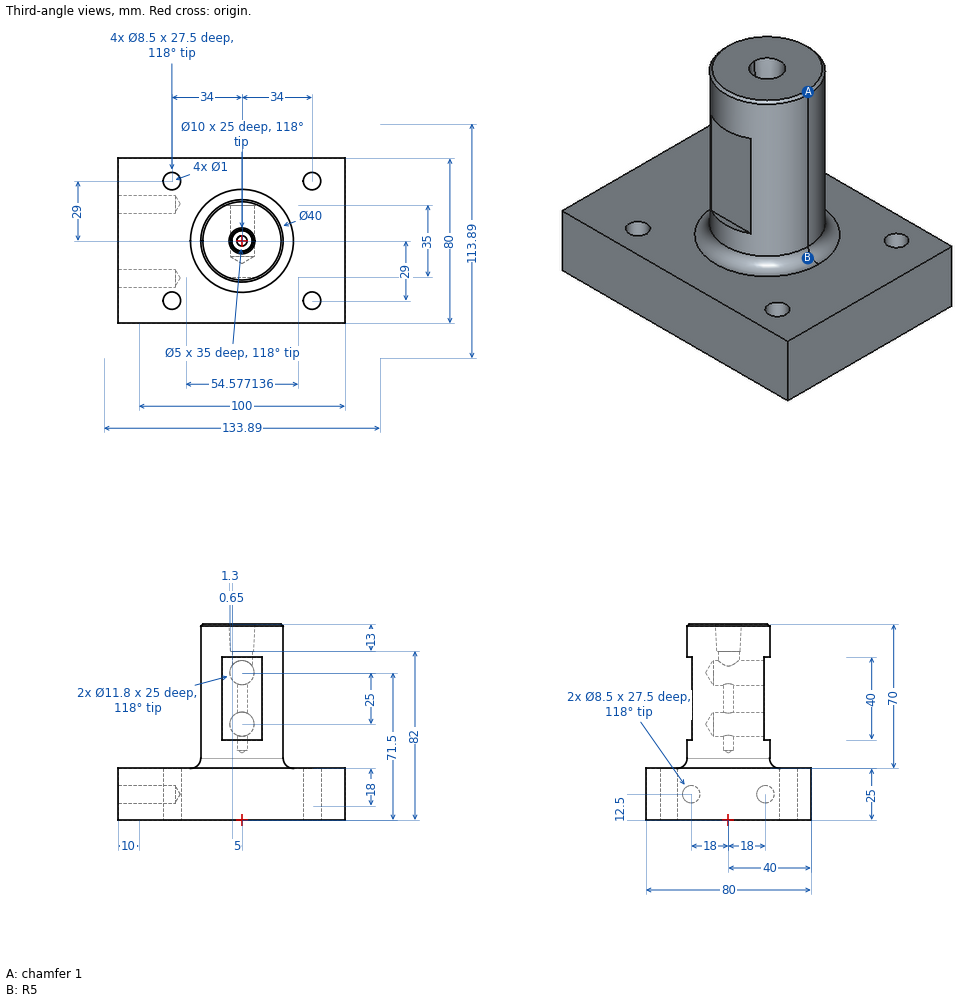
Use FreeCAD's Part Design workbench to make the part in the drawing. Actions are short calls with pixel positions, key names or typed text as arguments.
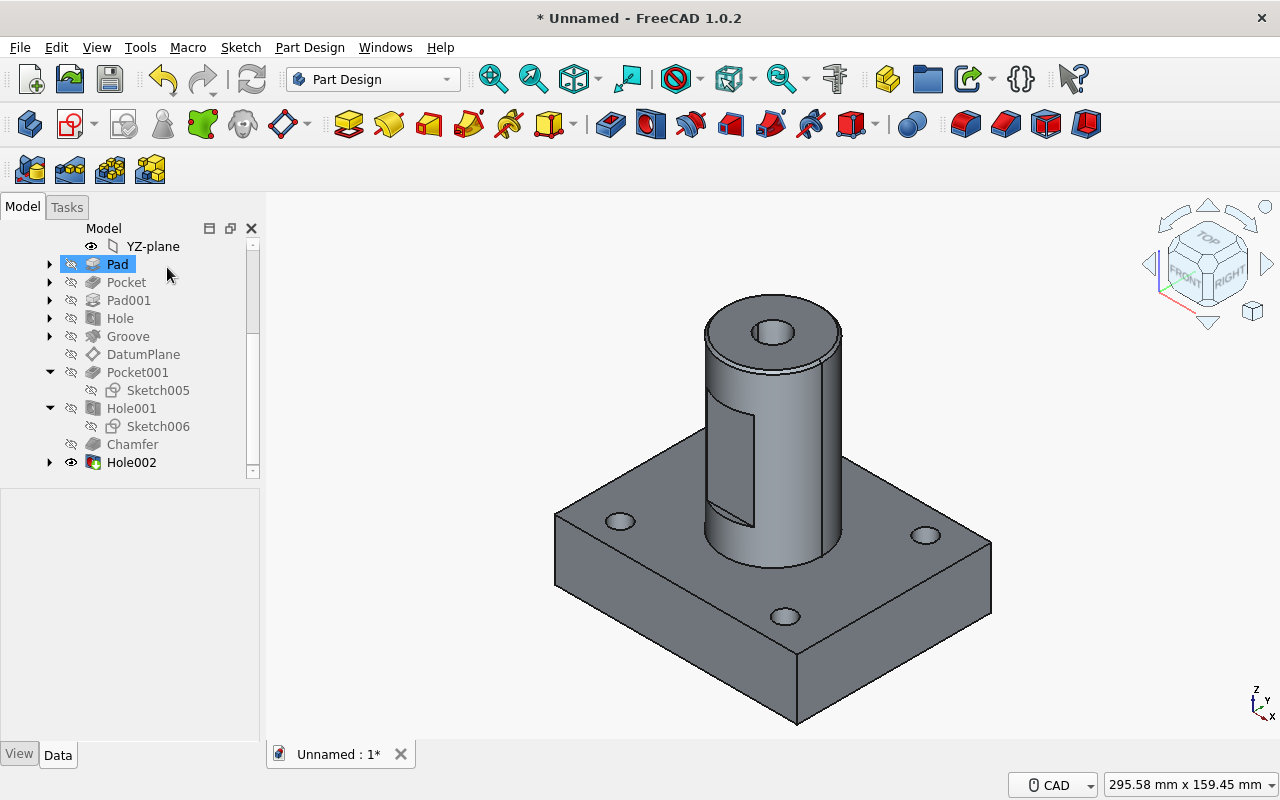
key(1)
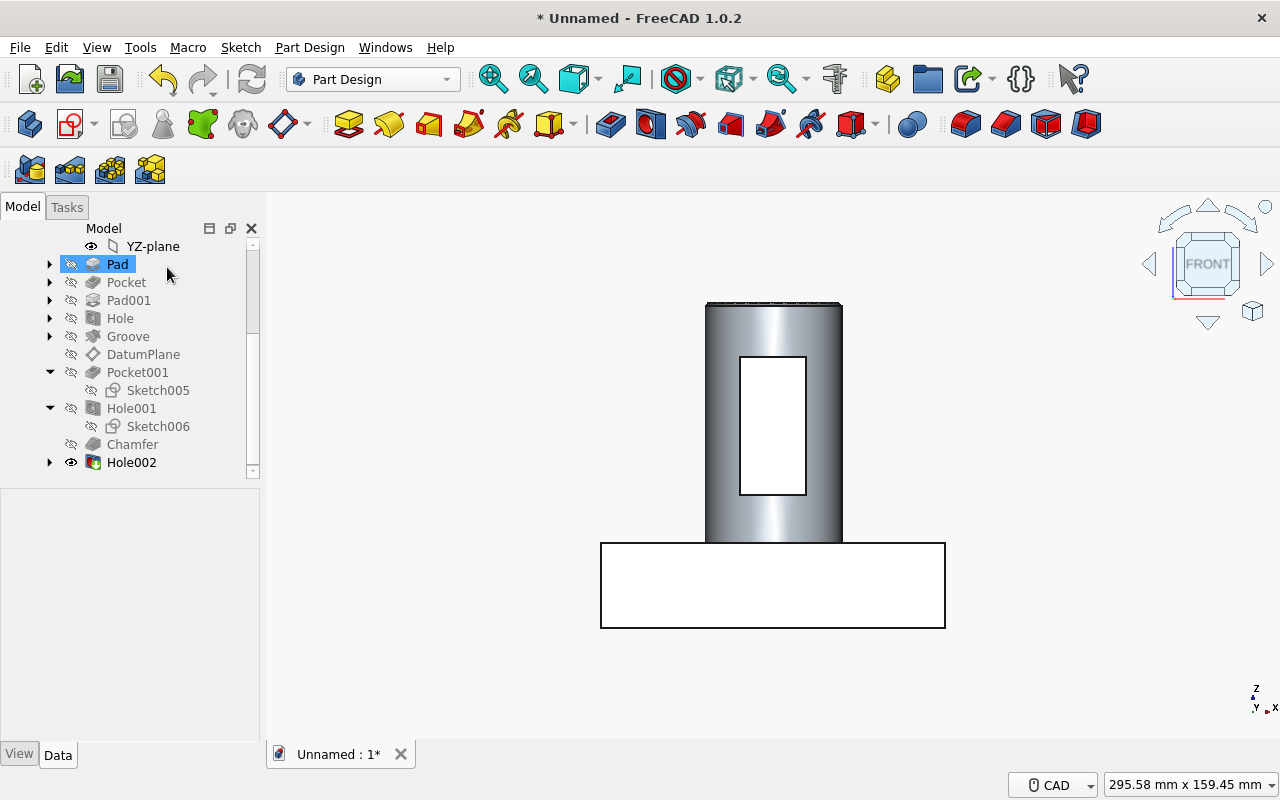
key(3)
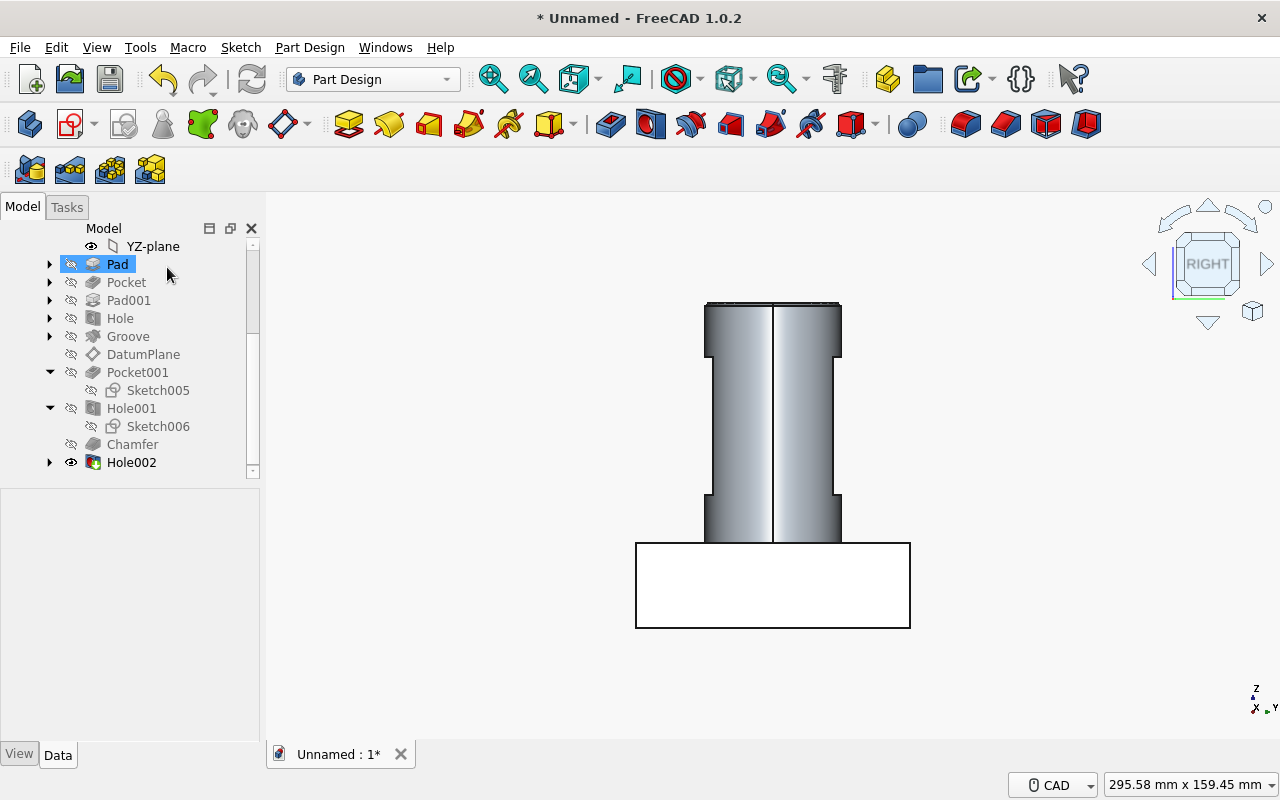
key(5)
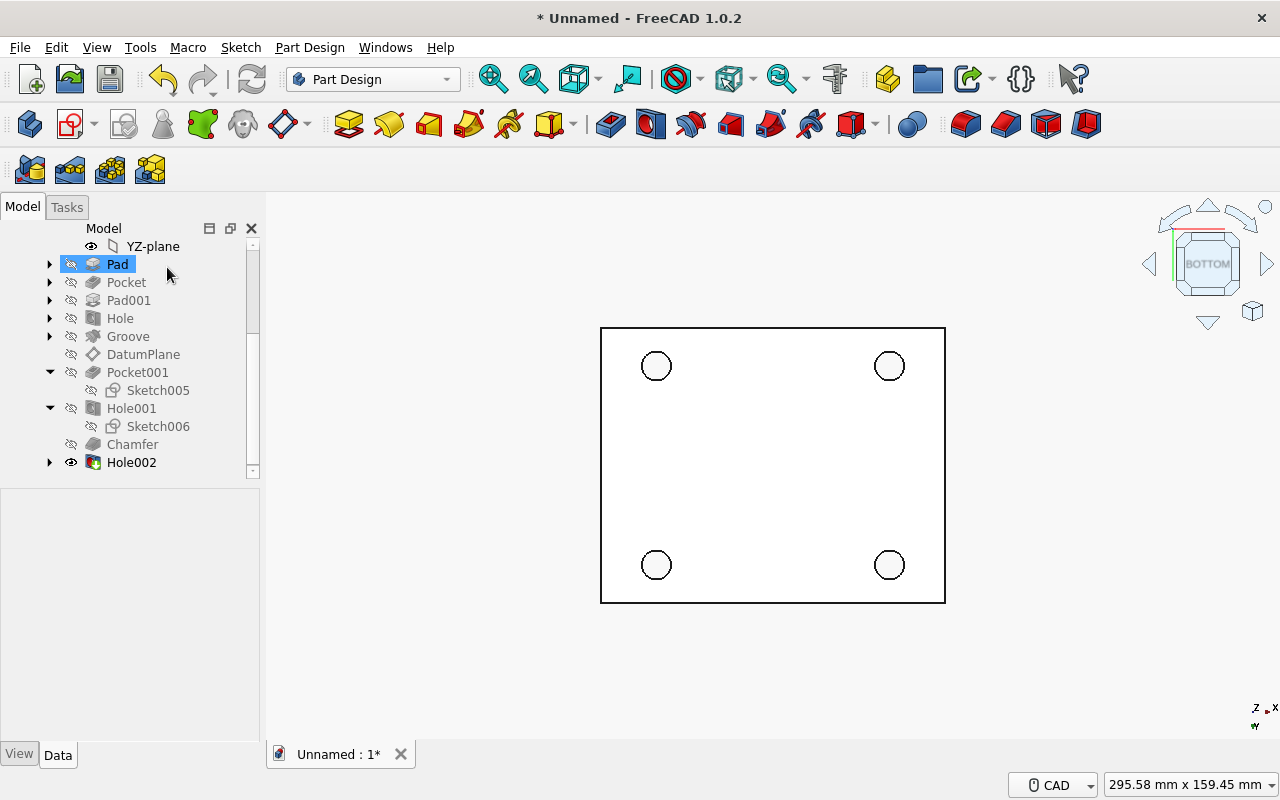
key(4)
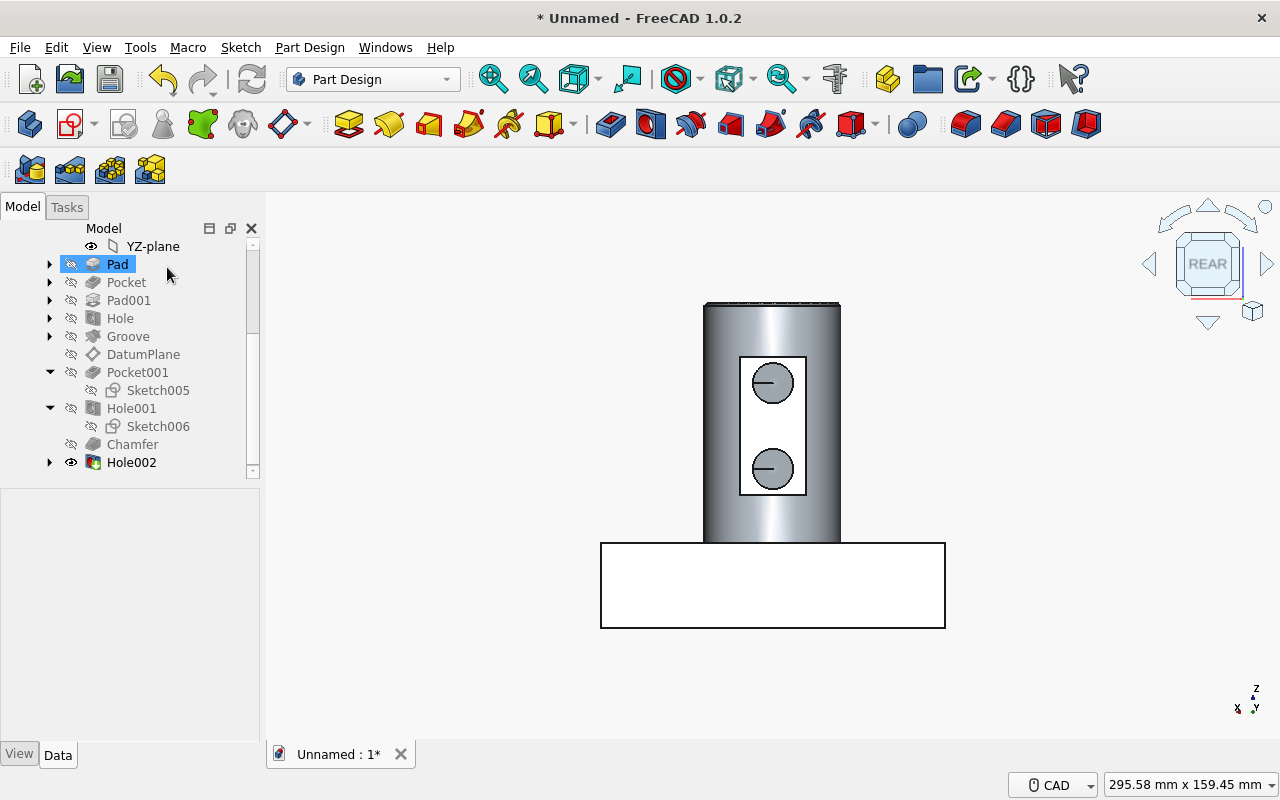
key(6)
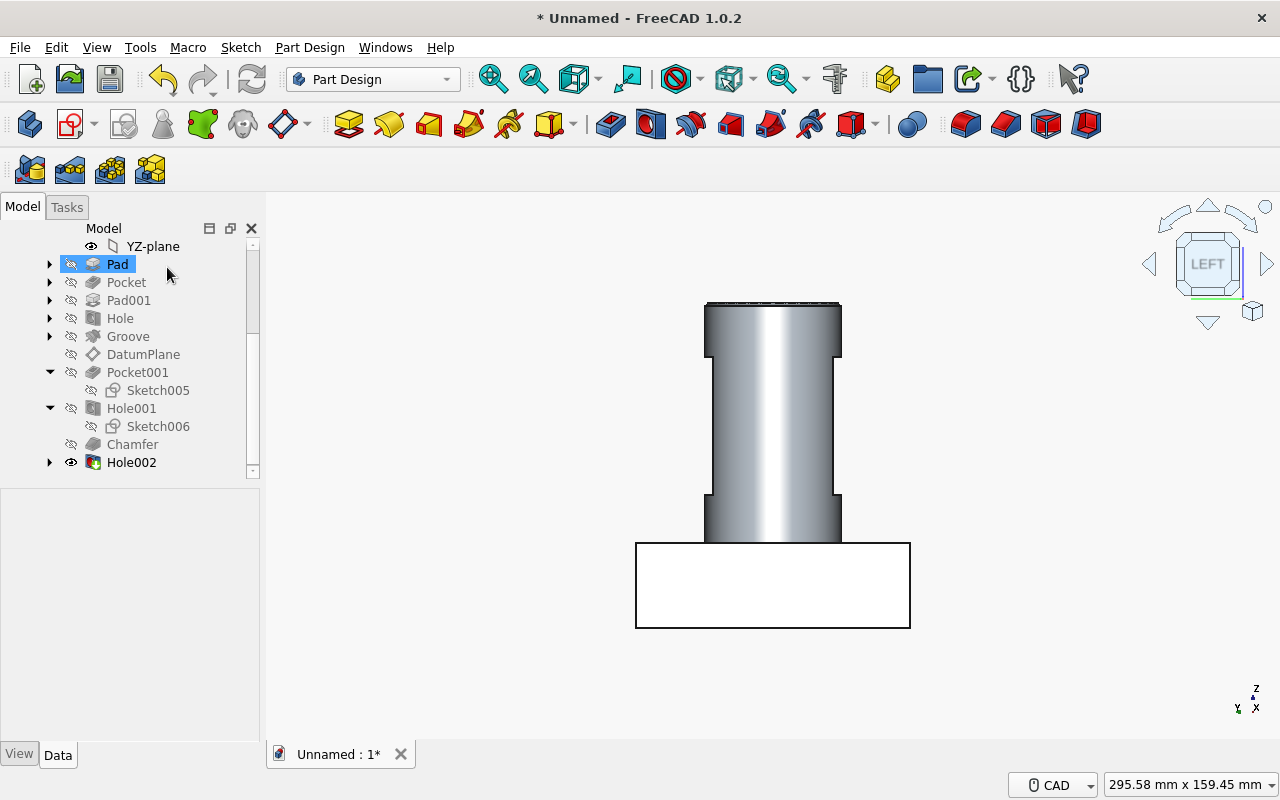
key(v)
key(3)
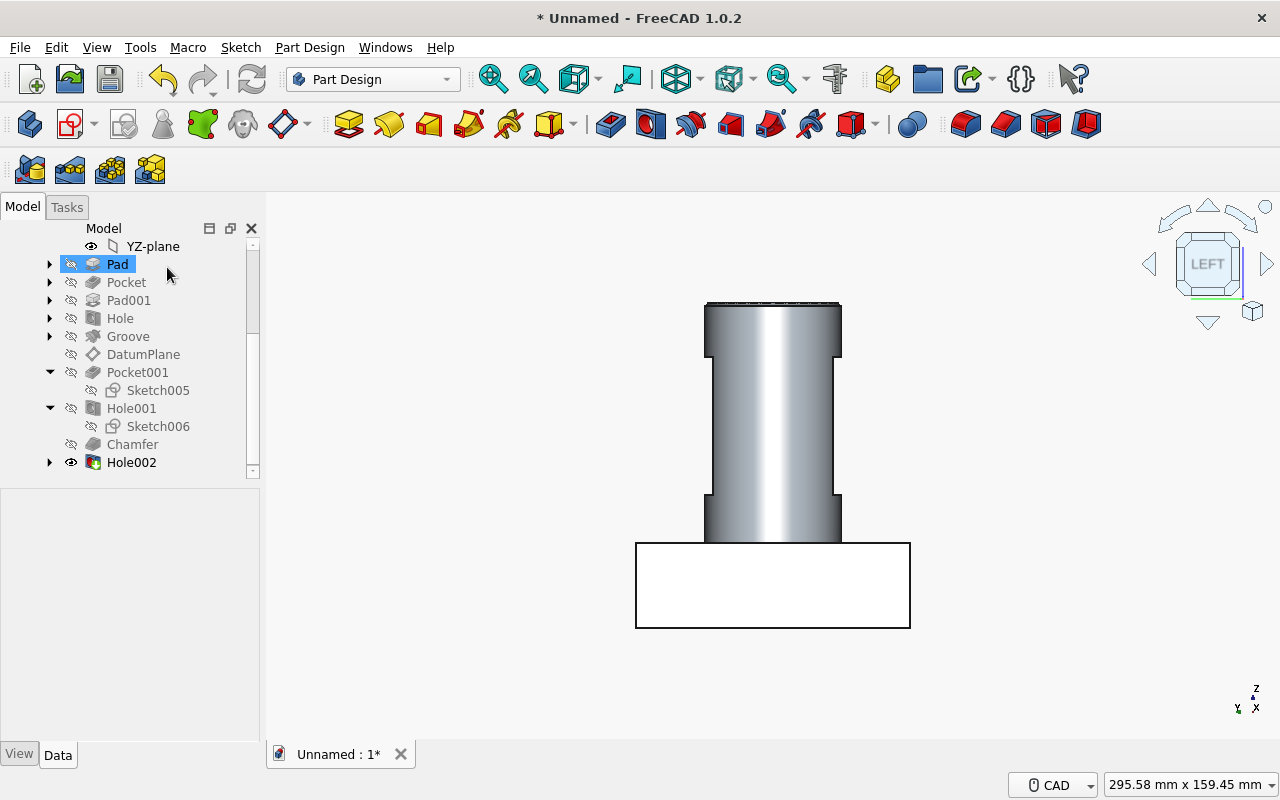
key(0)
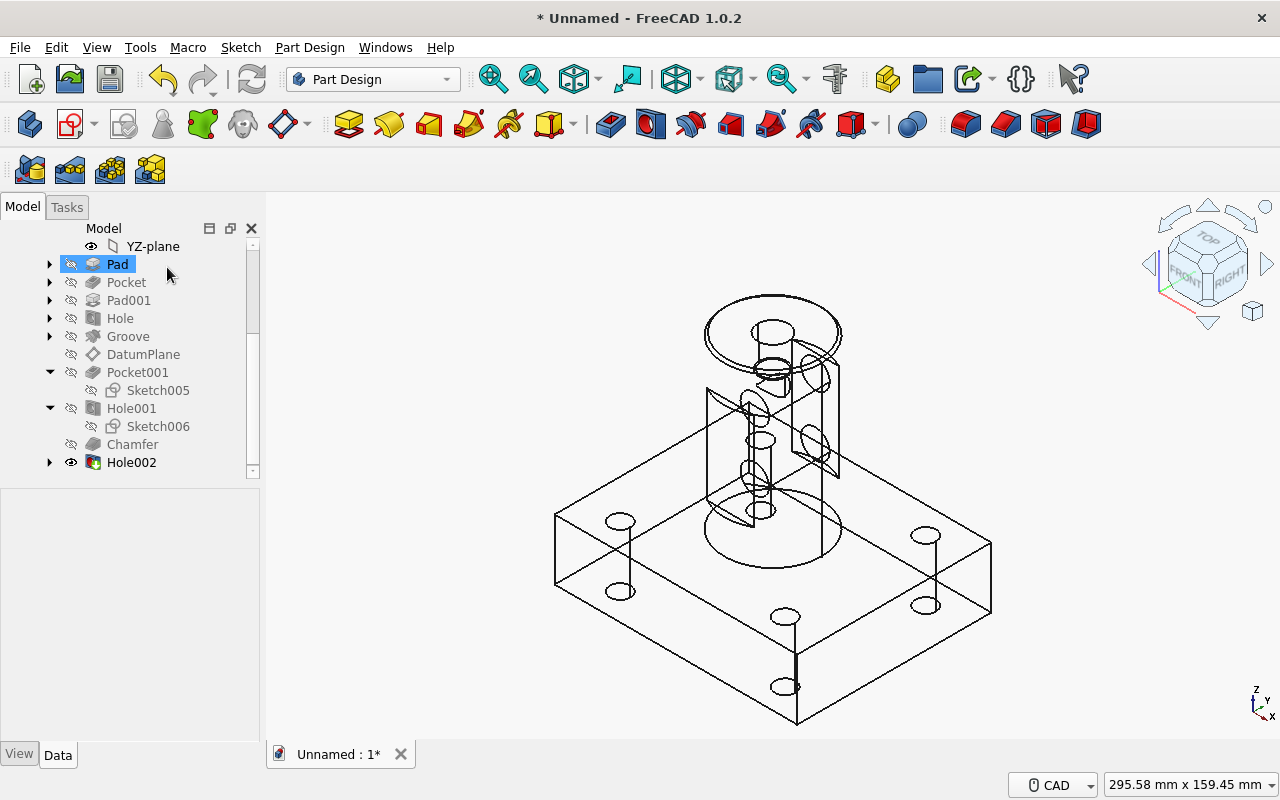
click(724, 500)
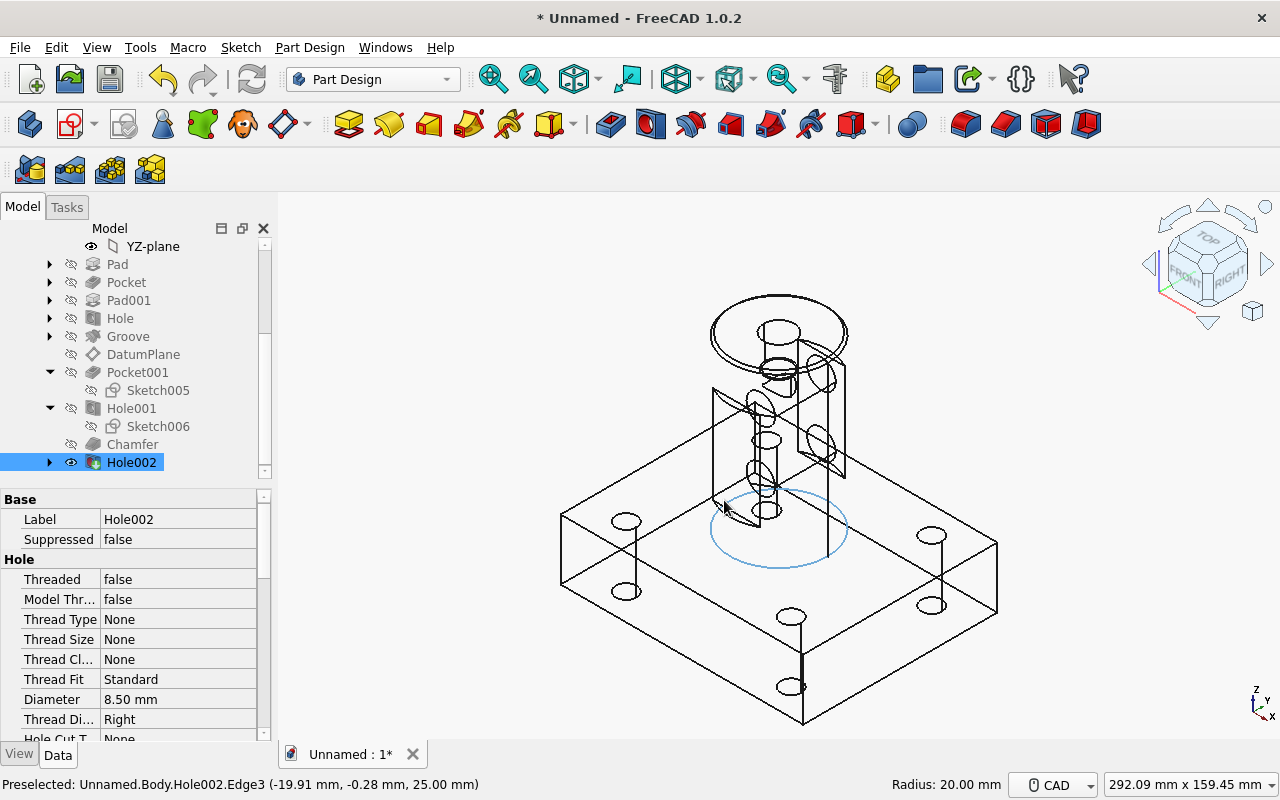
key(v)
key(1)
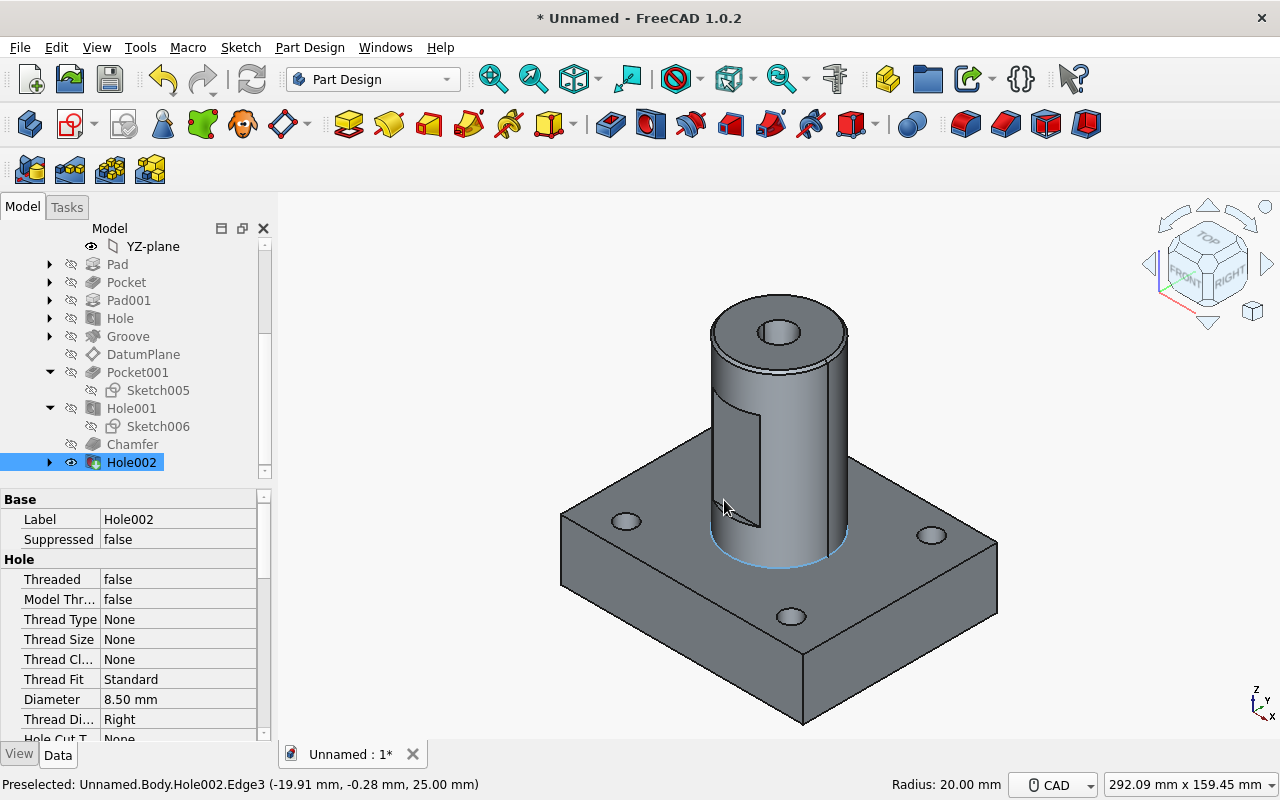
click(966, 124)